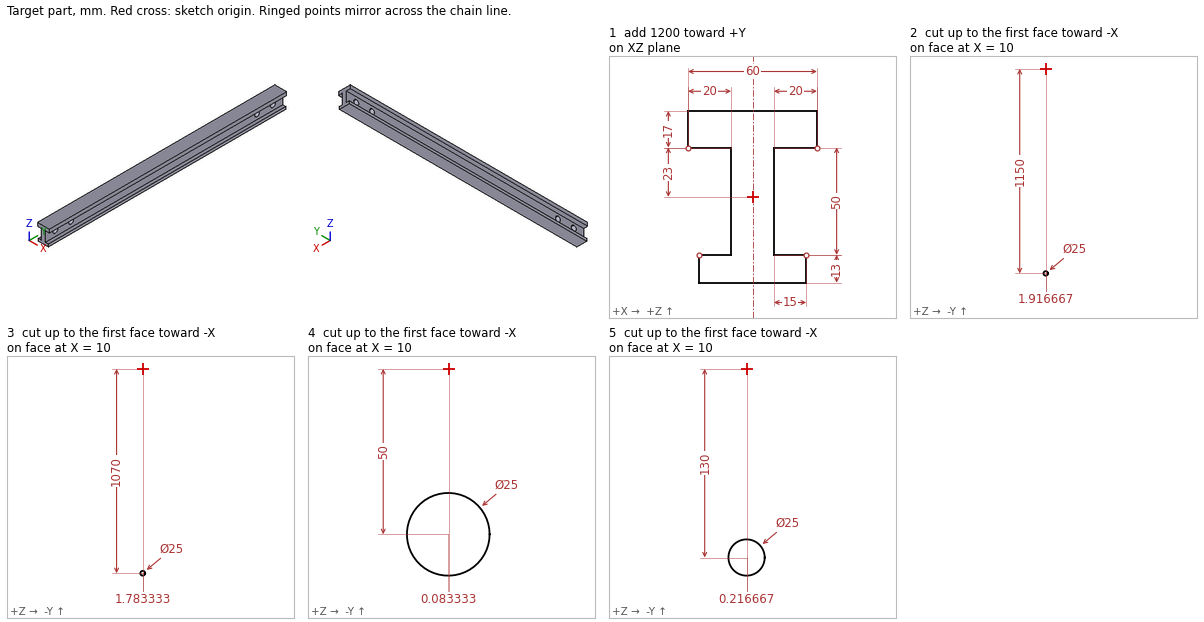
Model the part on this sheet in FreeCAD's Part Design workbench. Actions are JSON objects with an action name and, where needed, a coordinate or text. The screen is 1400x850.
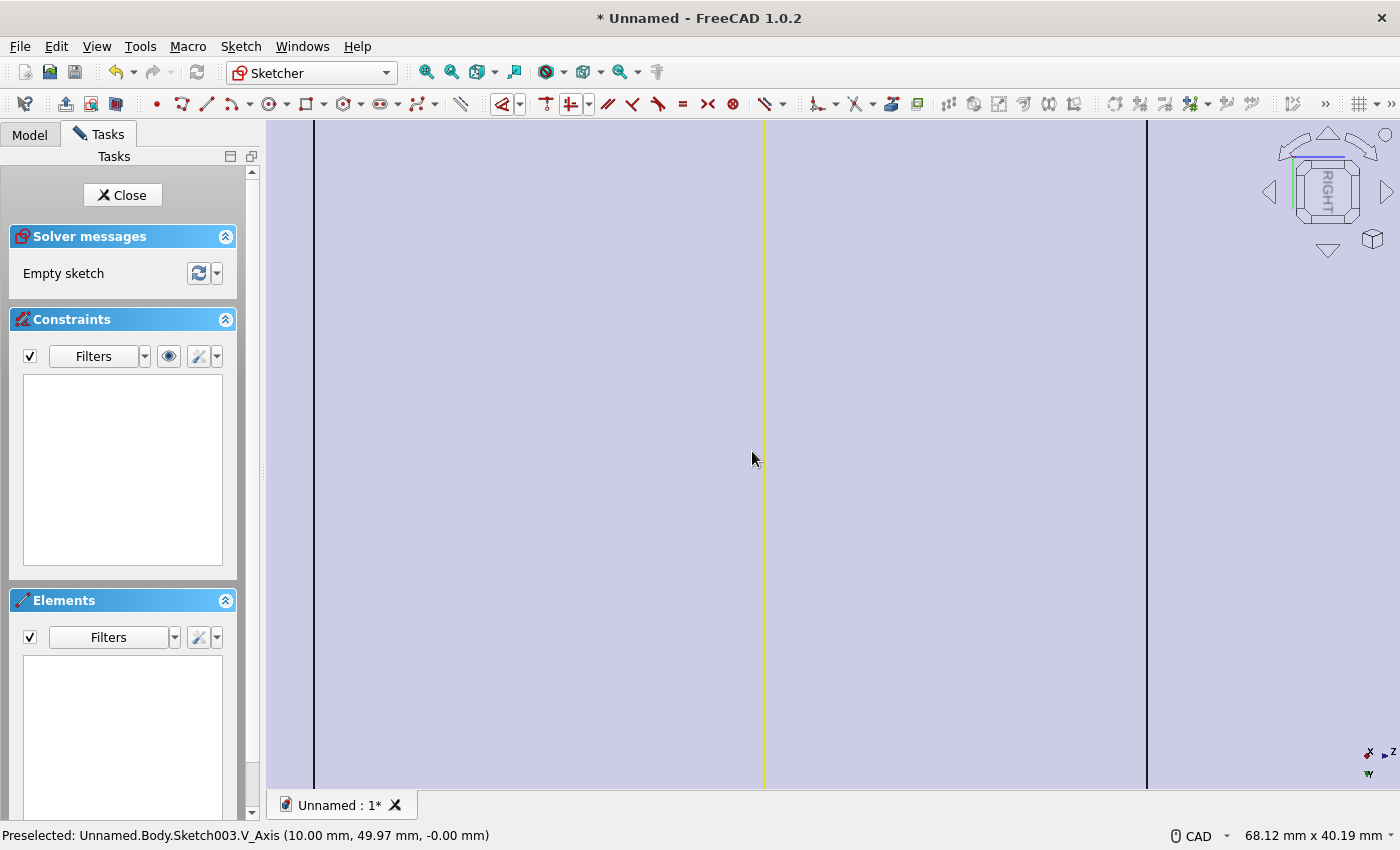
{"action": "left_click", "coordinate": [268, 104]}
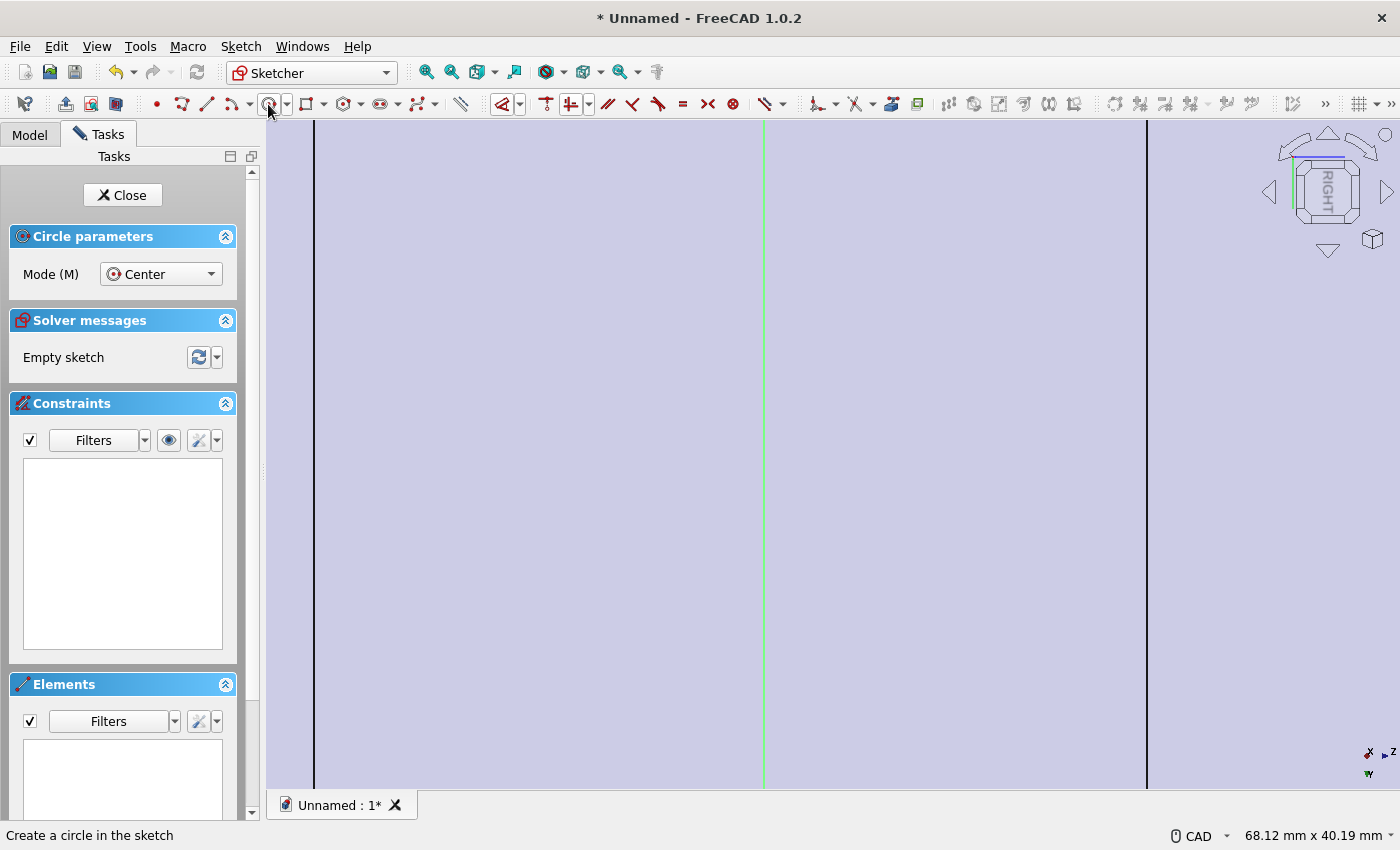
{"action": "scroll", "coordinate": [763, 454], "scroll_direction": "up", "scroll_amount": 13}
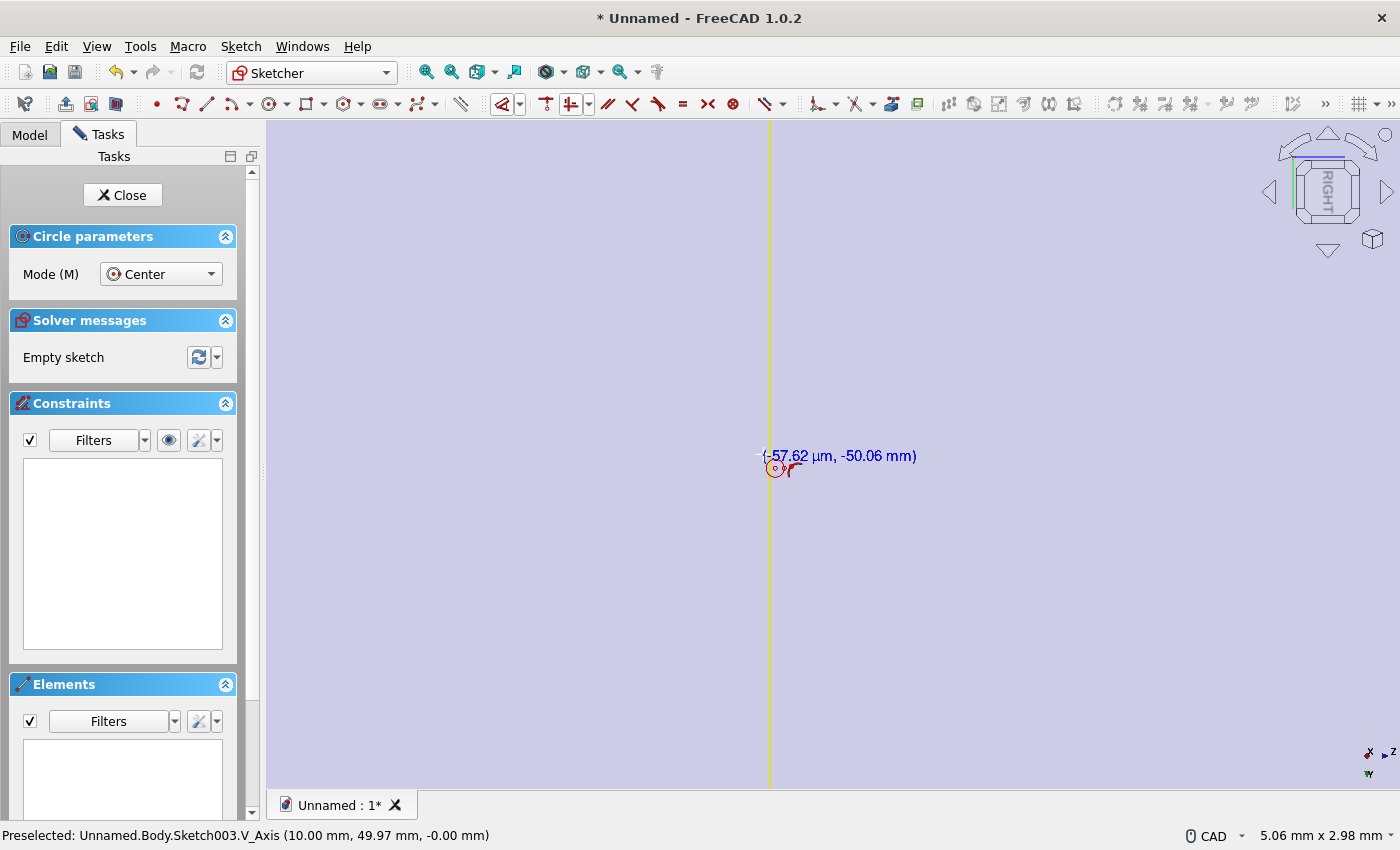
{"action": "left_click", "coordinate": [752, 448]}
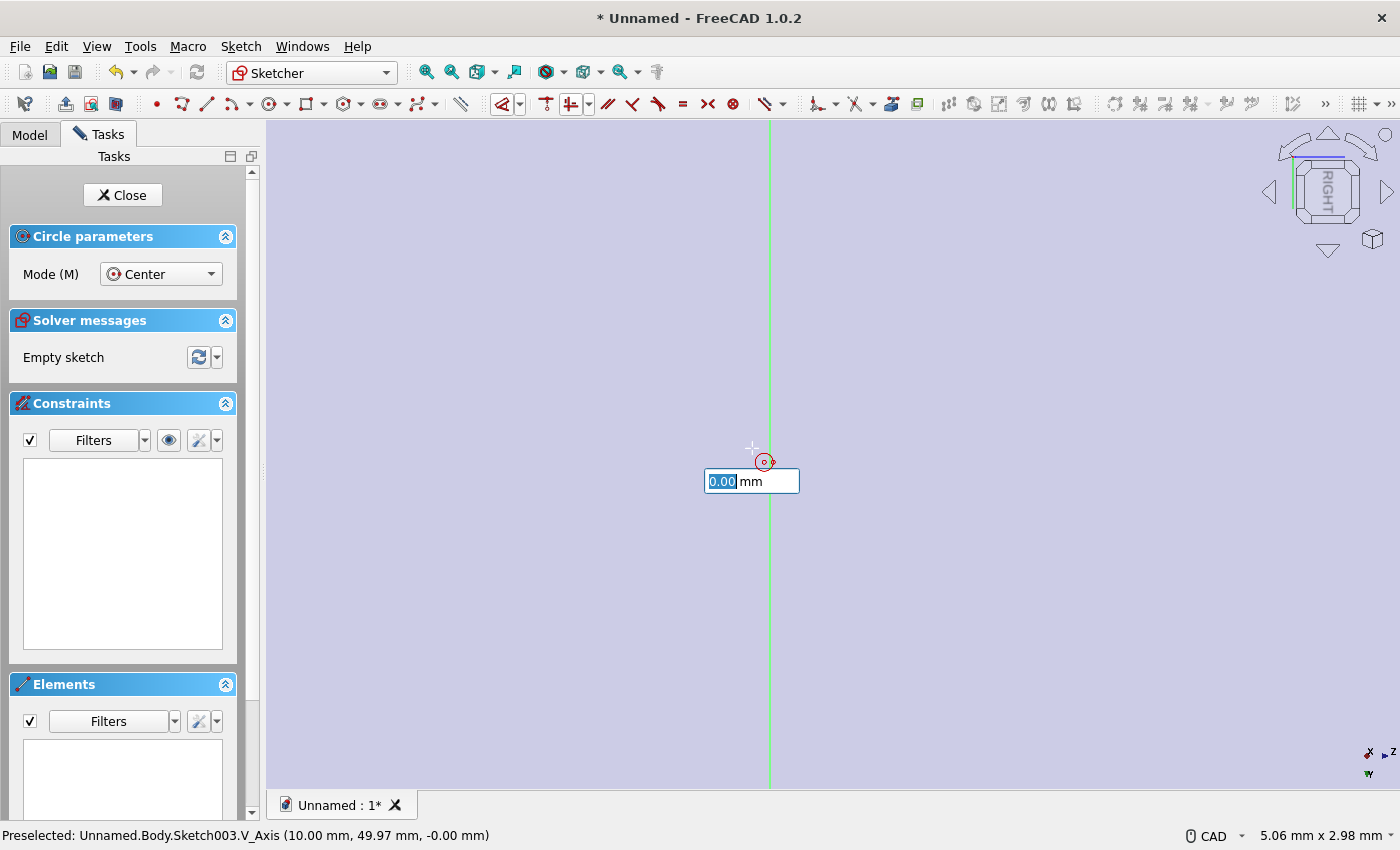
{"action": "scroll", "coordinate": [766, 455], "scroll_direction": "down", "scroll_amount": 13}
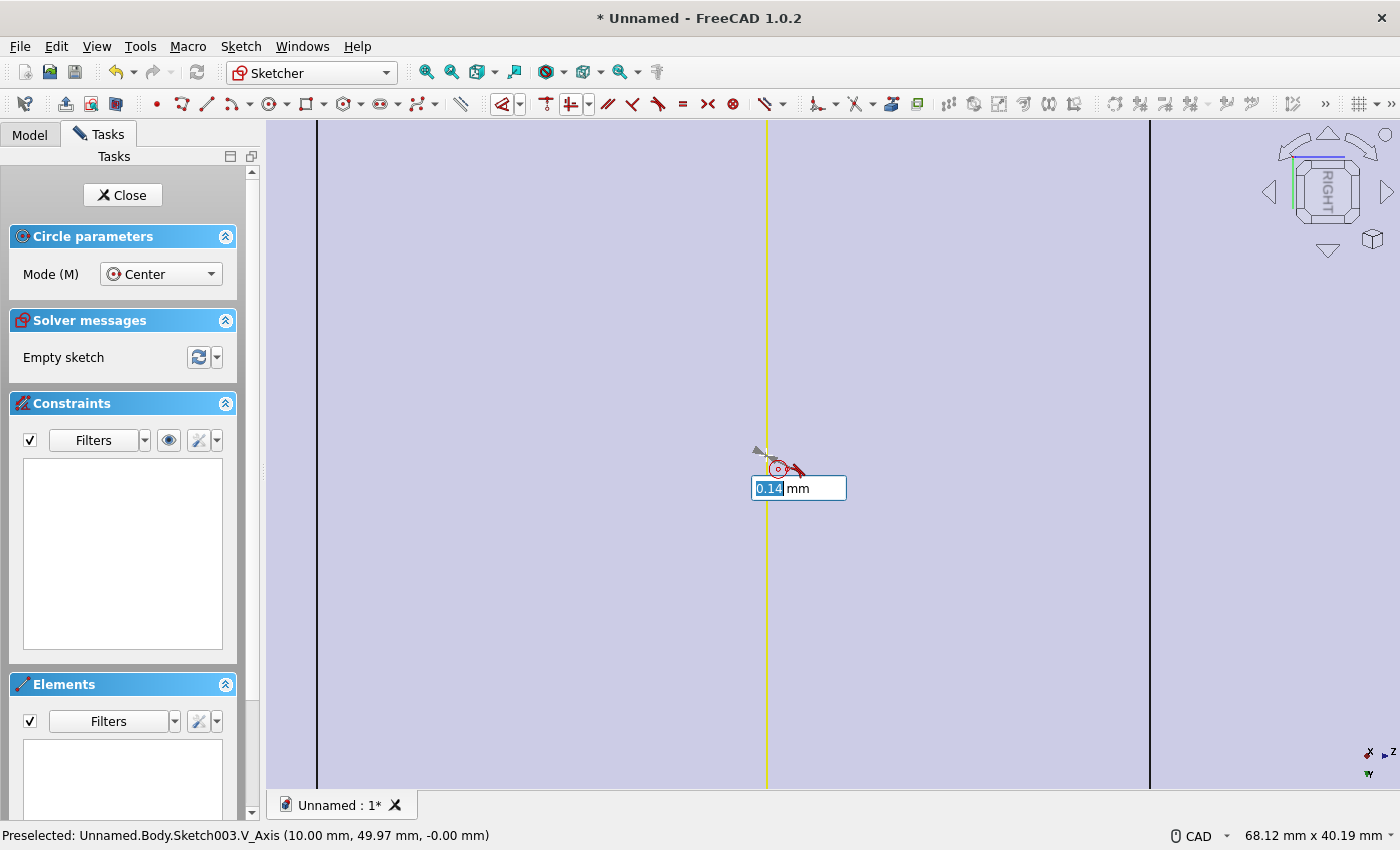
{"action": "left_click", "coordinate": [912, 308]}
{"action": "key", "text": "Escape"}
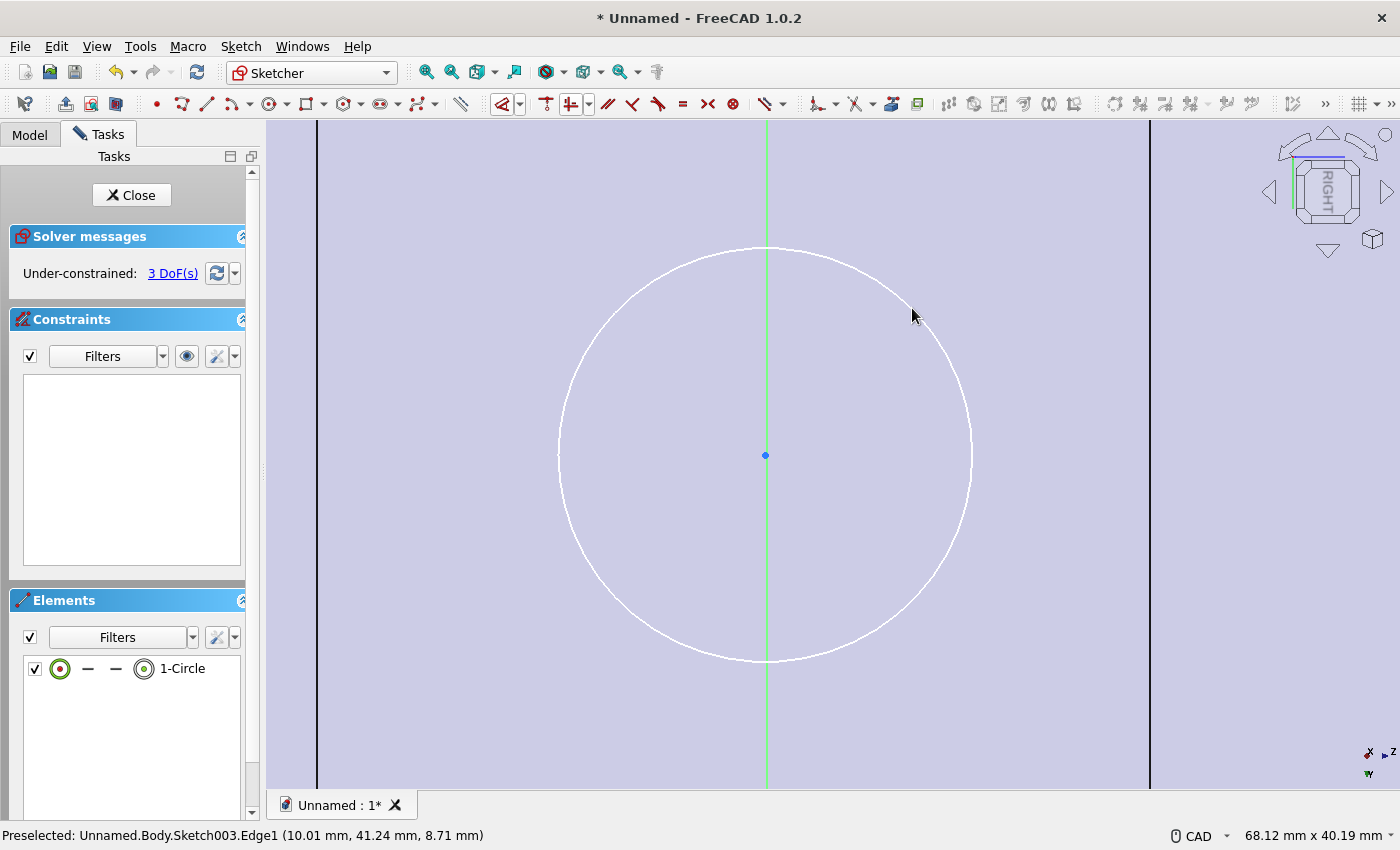
{"action": "left_click", "coordinate": [911, 308]}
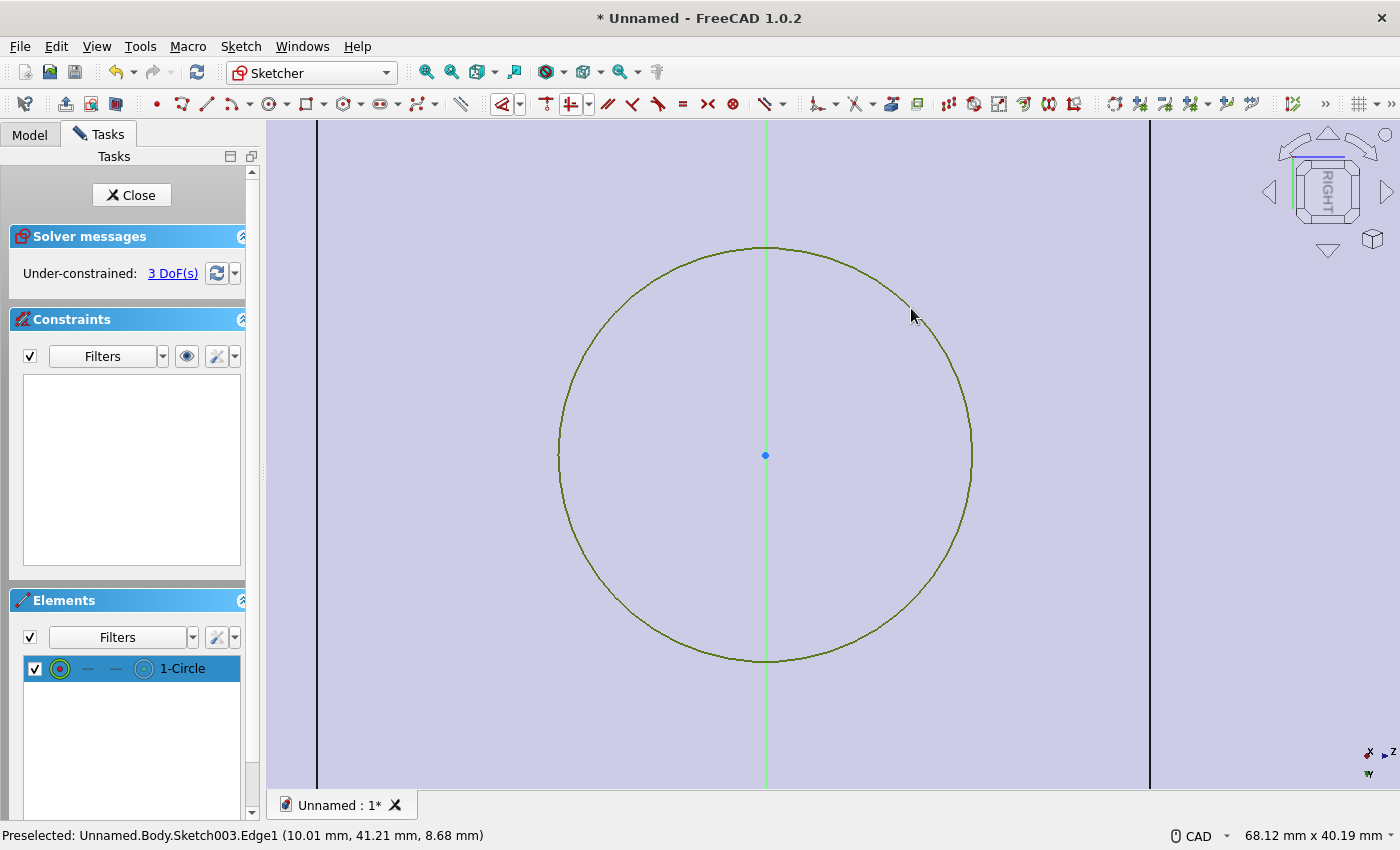
{"action": "left_click", "coordinate": [520, 104]}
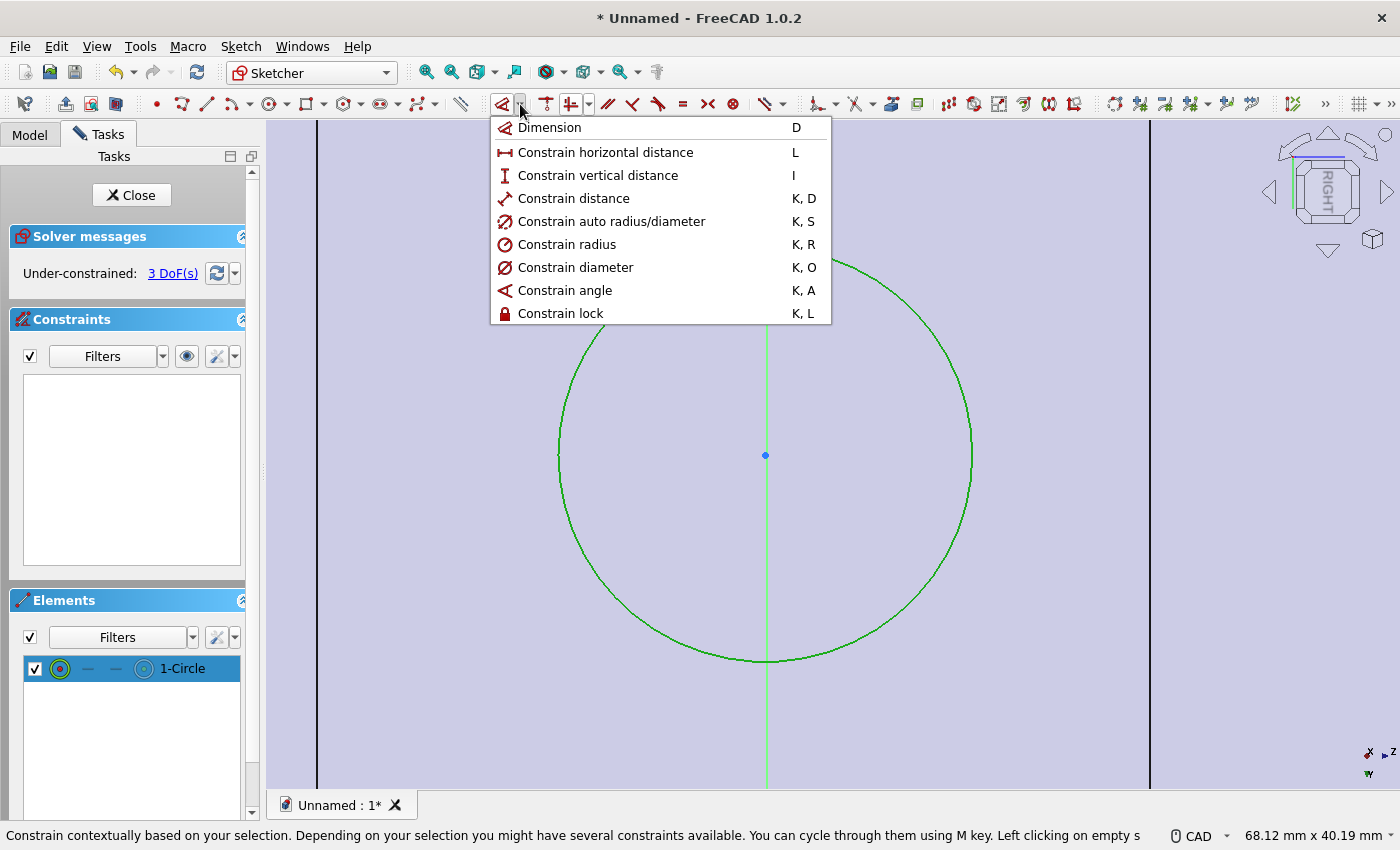
{"action": "left_click", "coordinate": [661, 268]}